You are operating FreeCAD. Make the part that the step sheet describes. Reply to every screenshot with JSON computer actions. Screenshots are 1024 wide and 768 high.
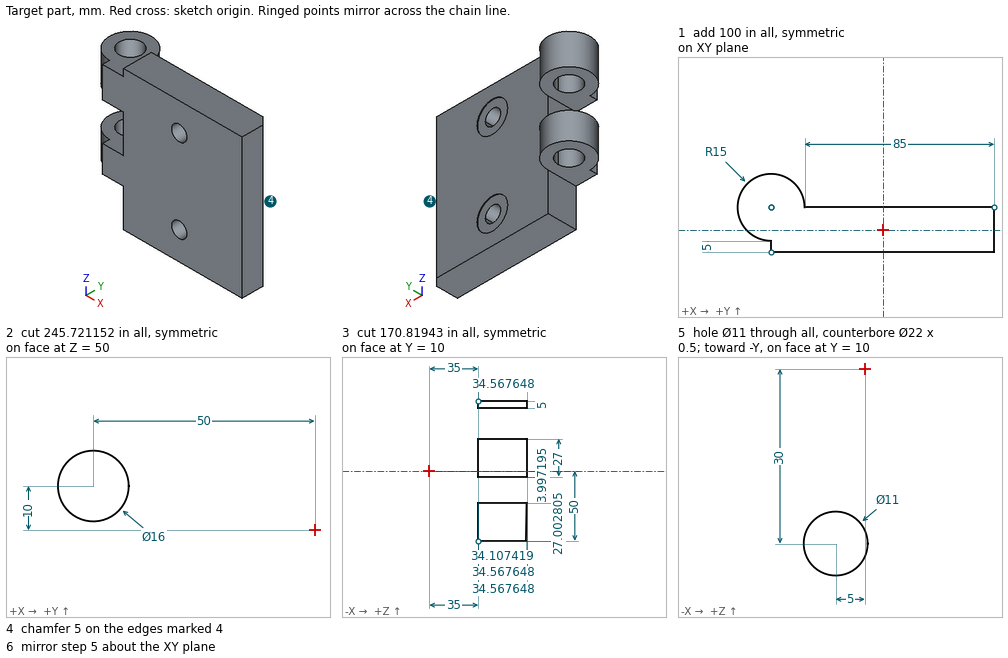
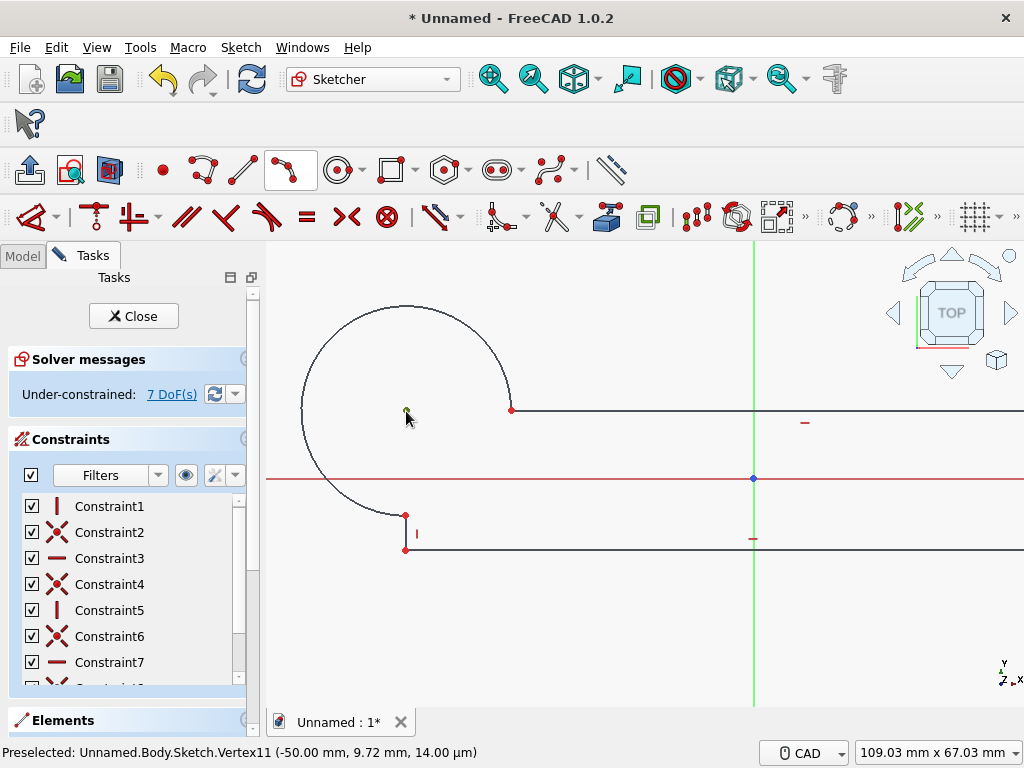
{"action": "left_click", "coordinate": [406, 550]}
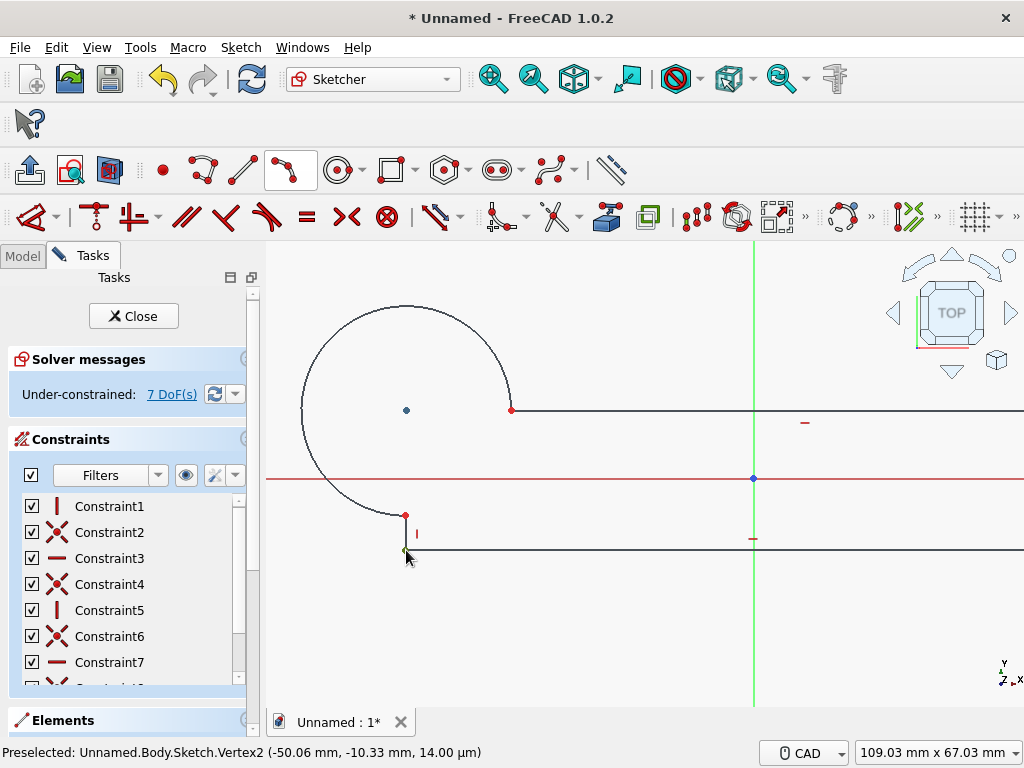
{"action": "left_click", "coordinate": [375, 479]}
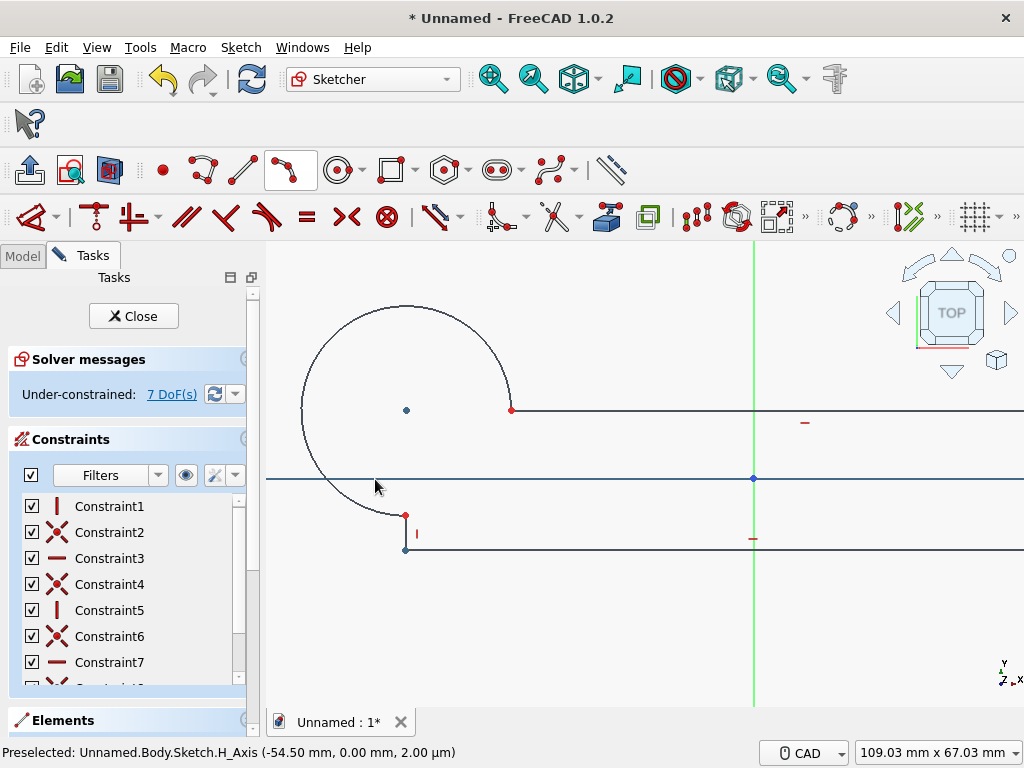
{"action": "left_click", "coordinate": [348, 218]}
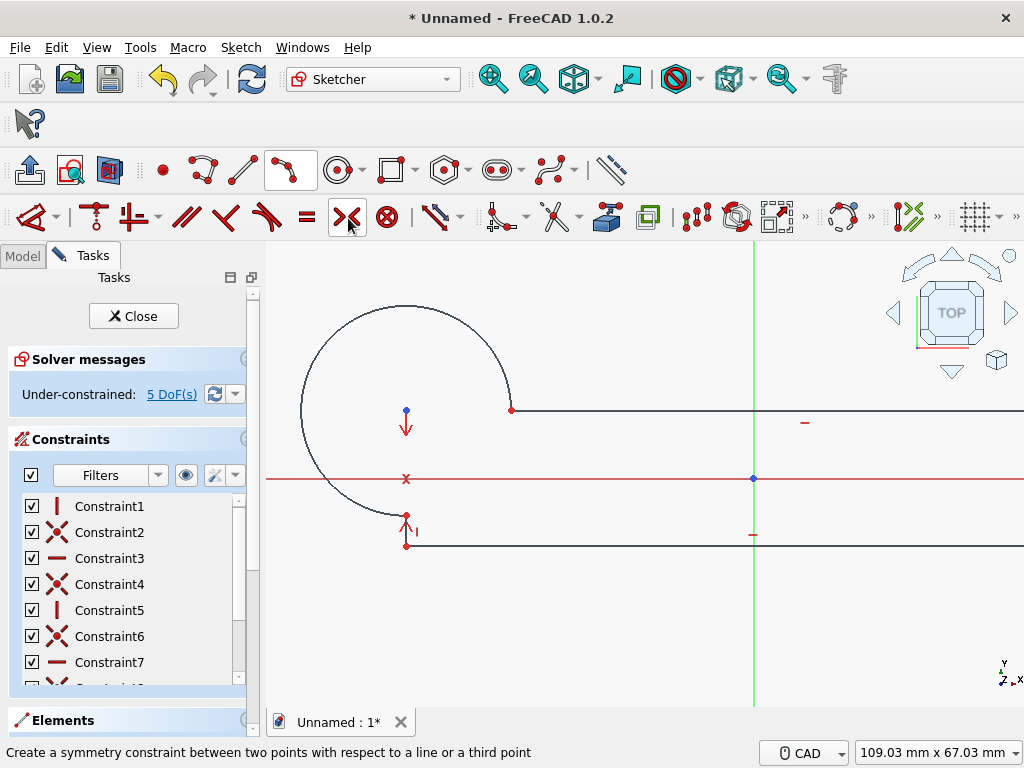
{"action": "left_click", "coordinate": [406, 411]}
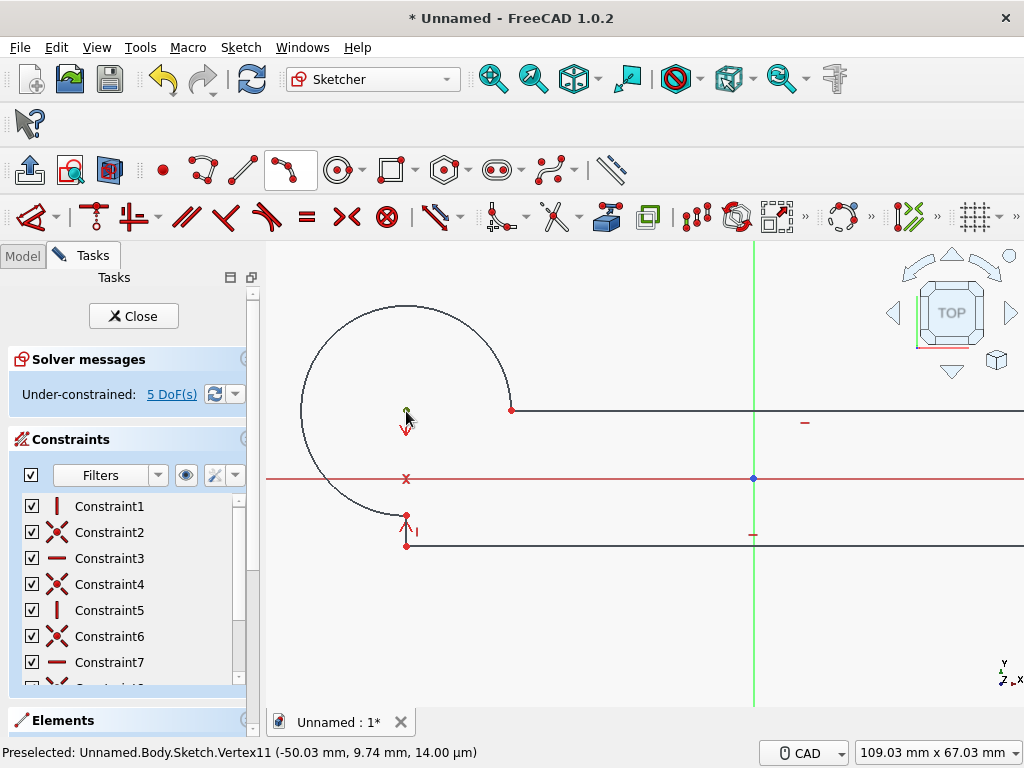
{"action": "scroll", "coordinate": [406, 513], "scroll_direction": "down", "scroll_amount": 3}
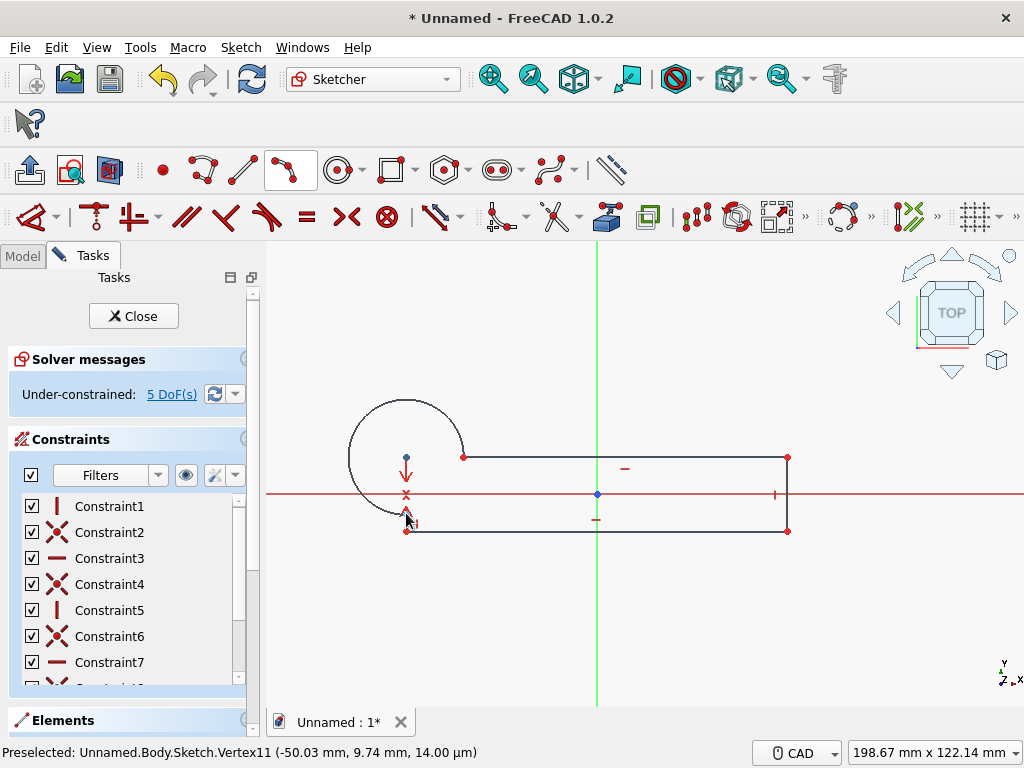
{"action": "left_click", "coordinate": [787, 457]}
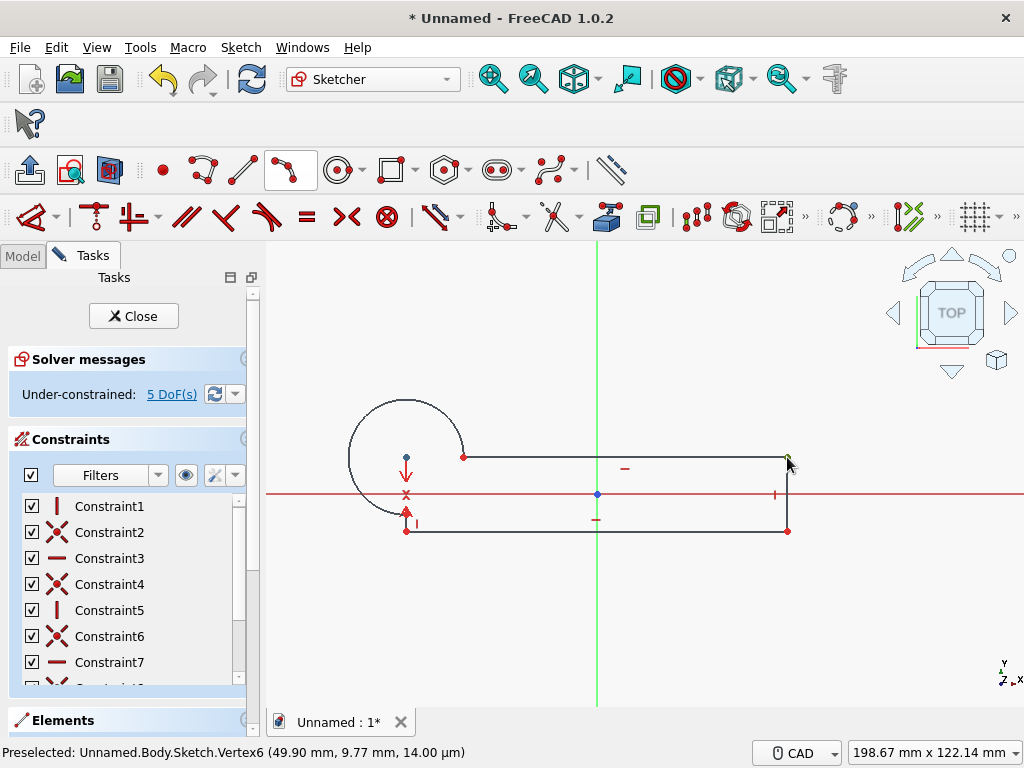
{"action": "left_click", "coordinate": [597, 650]}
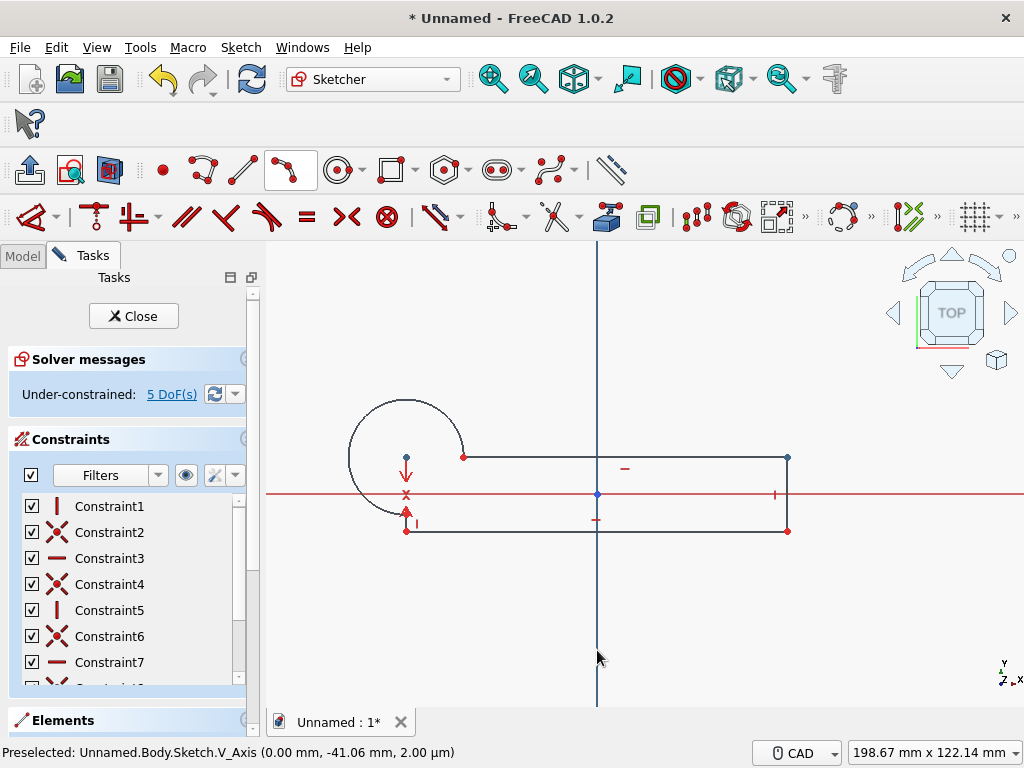
{"action": "left_click", "coordinate": [348, 218]}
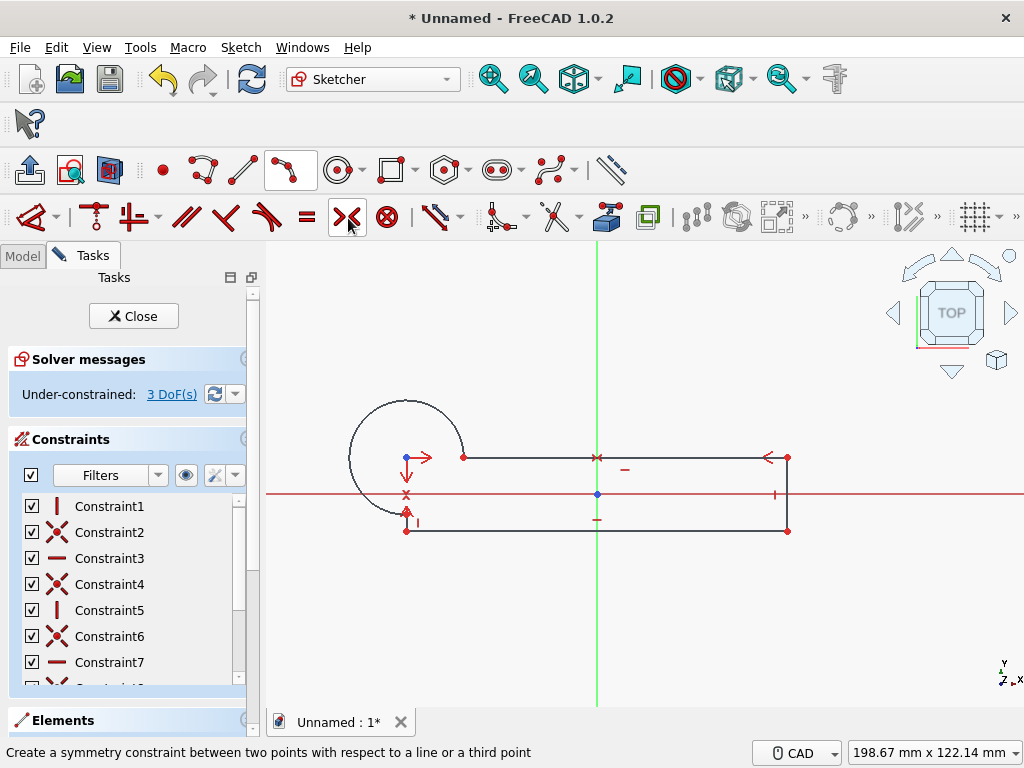
{"action": "left_click", "coordinate": [416, 401]}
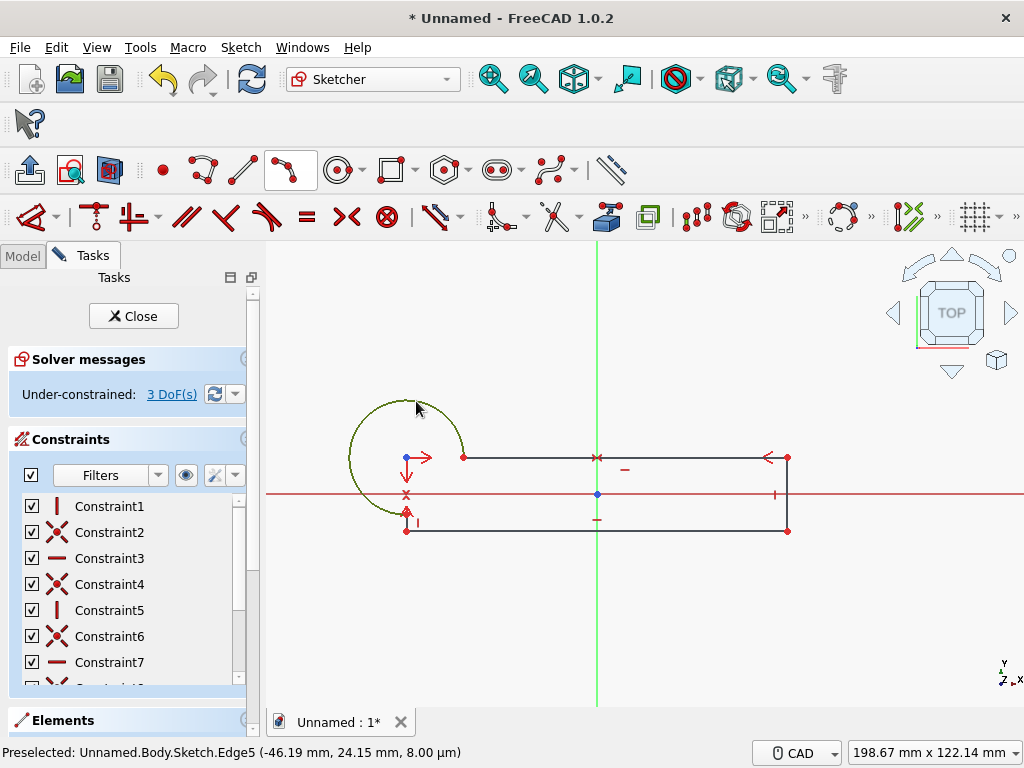
{"action": "left_click", "coordinate": [58, 218]}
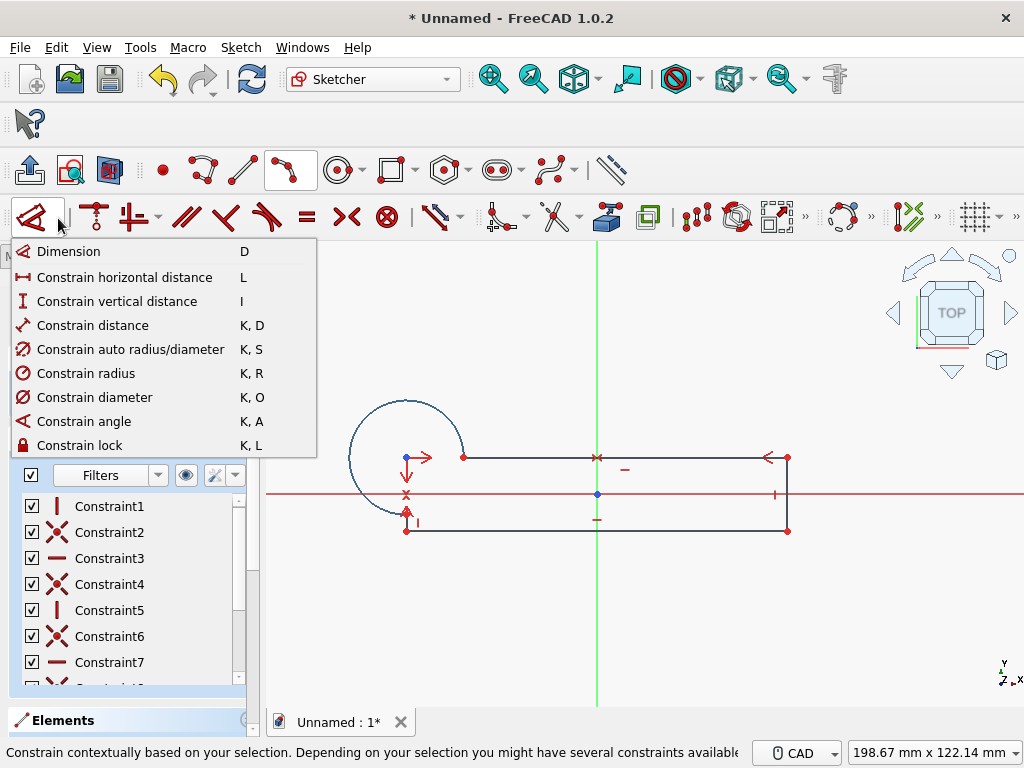
{"action": "left_click", "coordinate": [164, 373]}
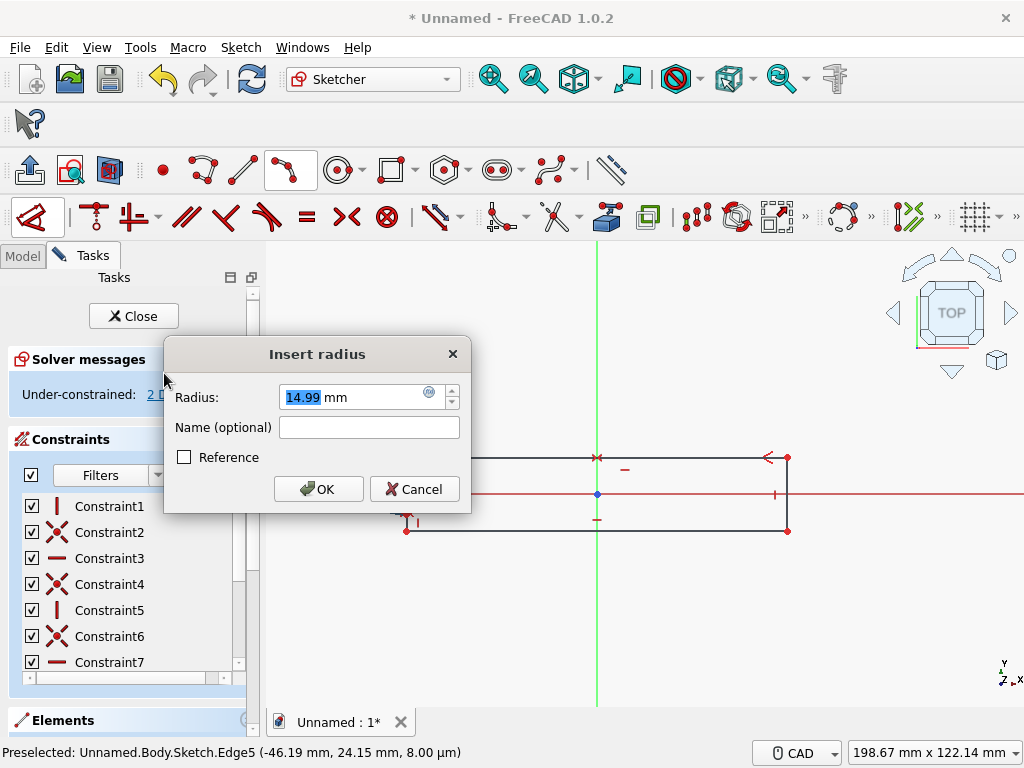
{"action": "type", "text": "15"}
{"action": "key", "text": "Return"}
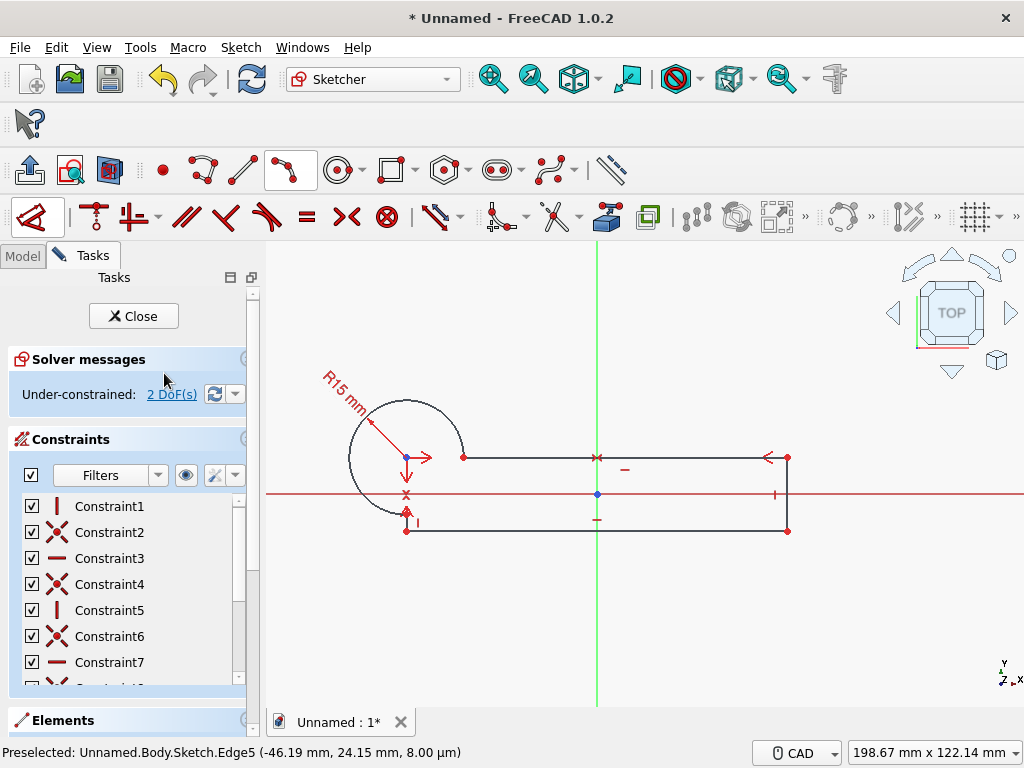
{"action": "scroll", "coordinate": [407, 523], "scroll_direction": "up", "scroll_amount": 4}